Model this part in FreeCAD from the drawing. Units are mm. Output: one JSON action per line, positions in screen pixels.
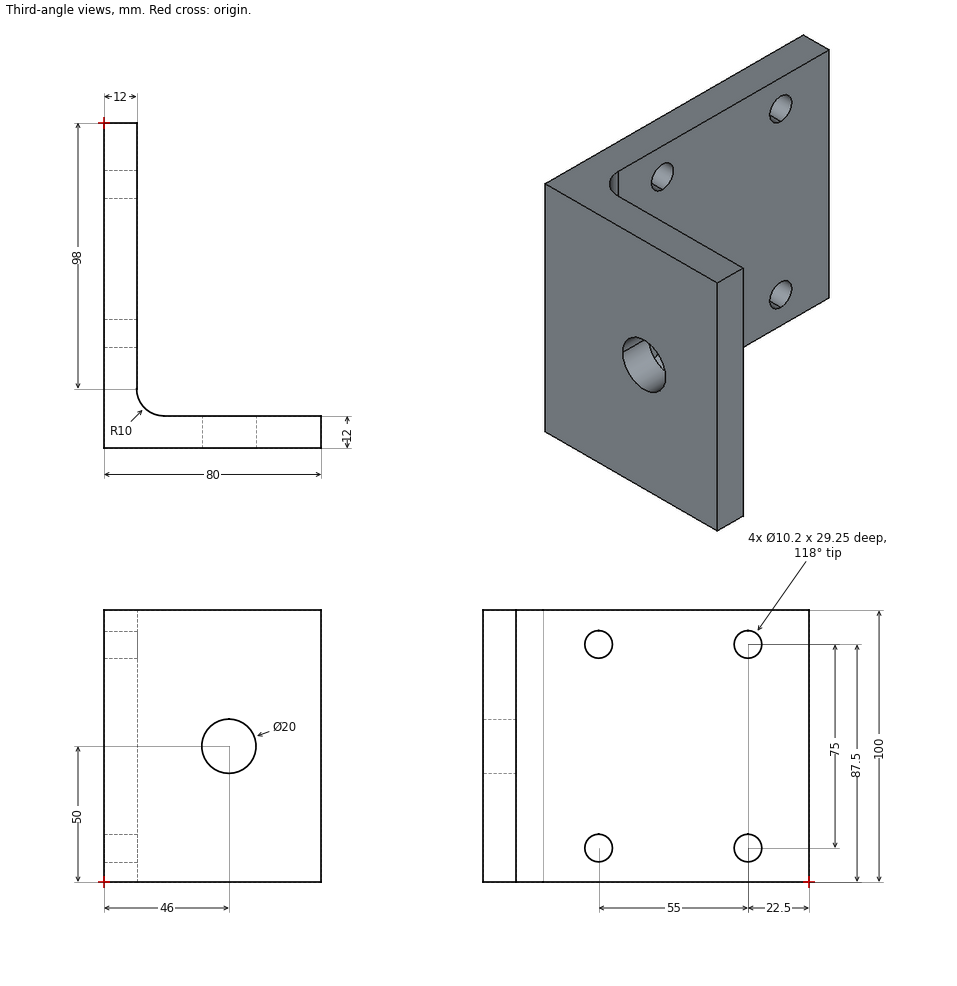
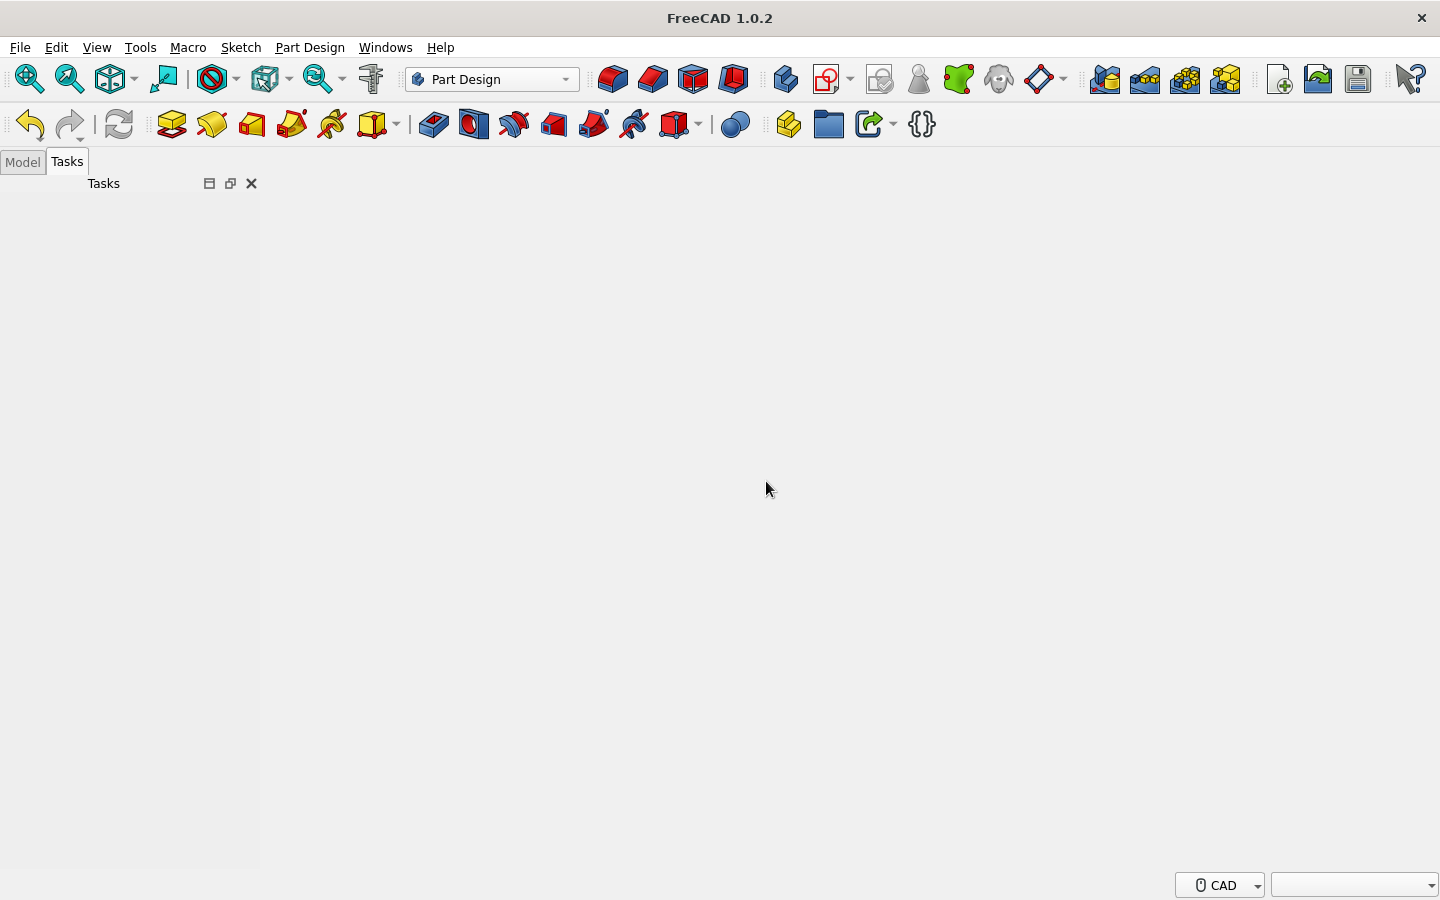
{"action": "left_click", "coordinate": [1278, 80]}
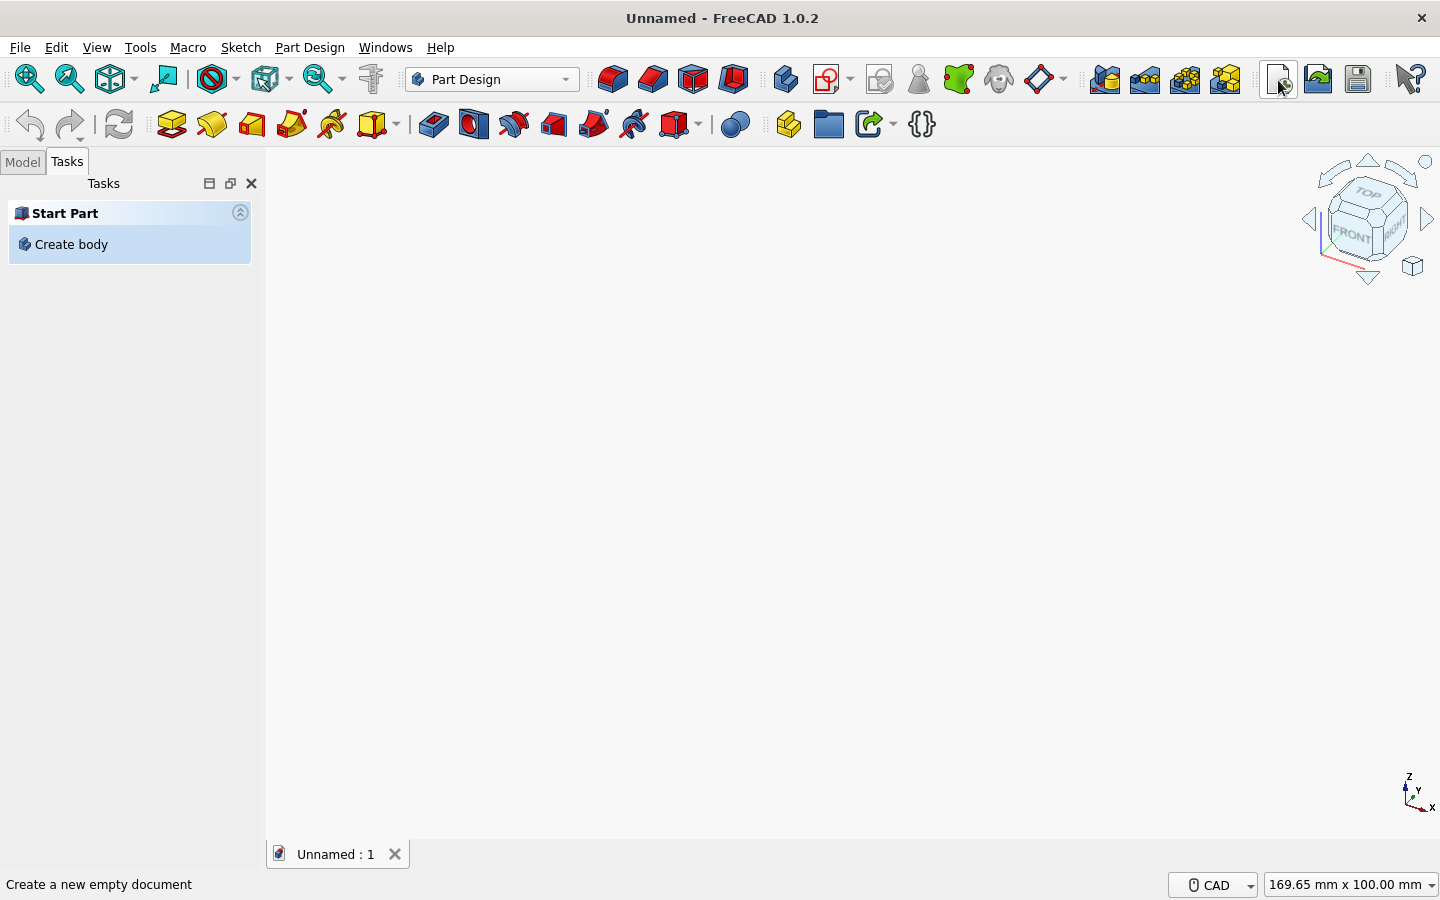
{"action": "left_click", "coordinate": [826, 80]}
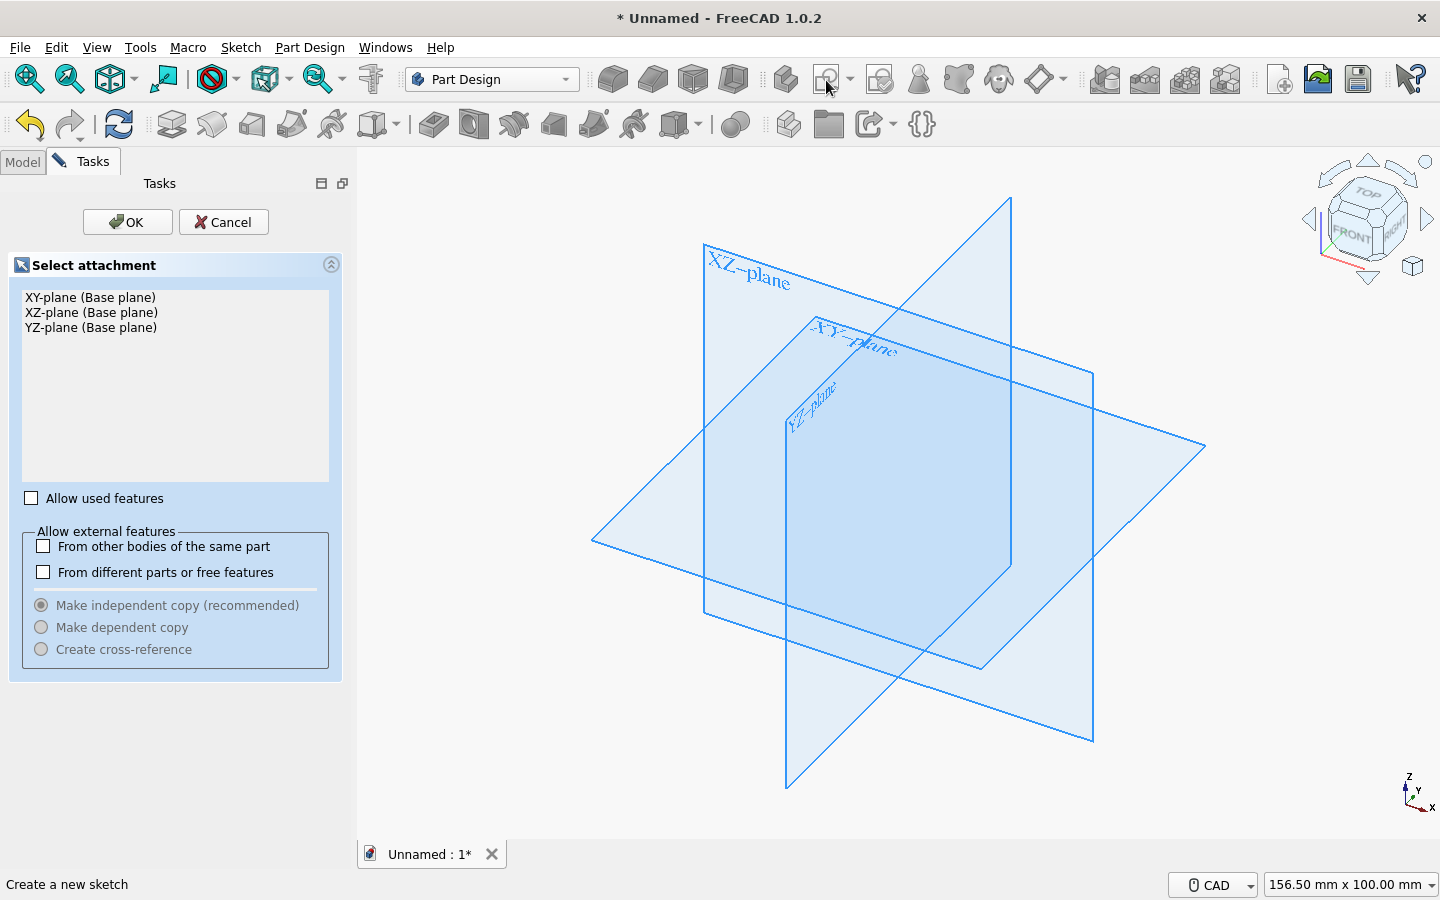
{"action": "left_click", "coordinate": [82, 298]}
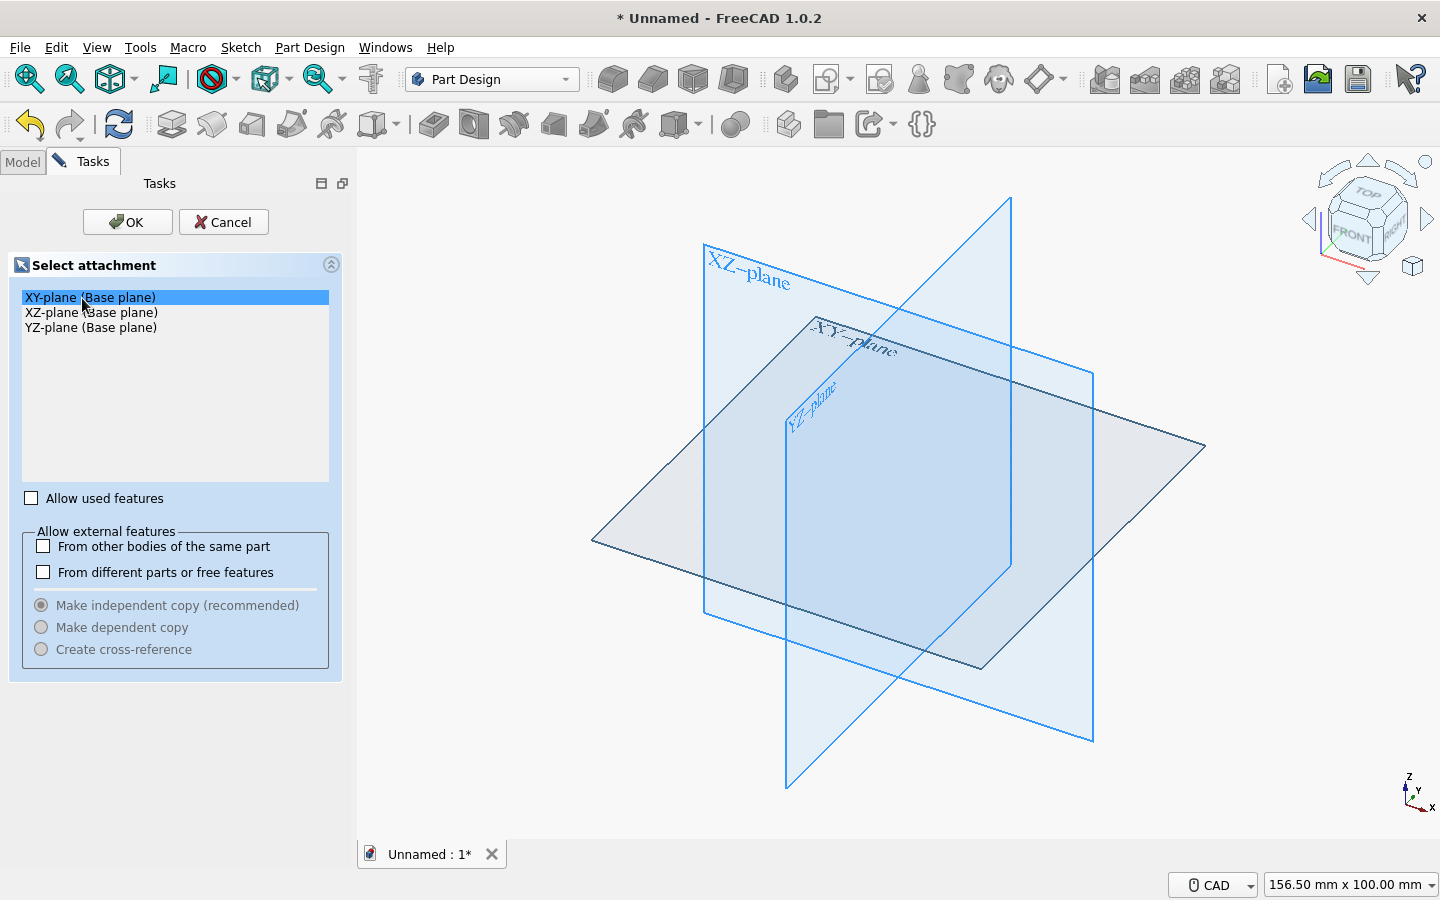
{"action": "left_click", "coordinate": [128, 222]}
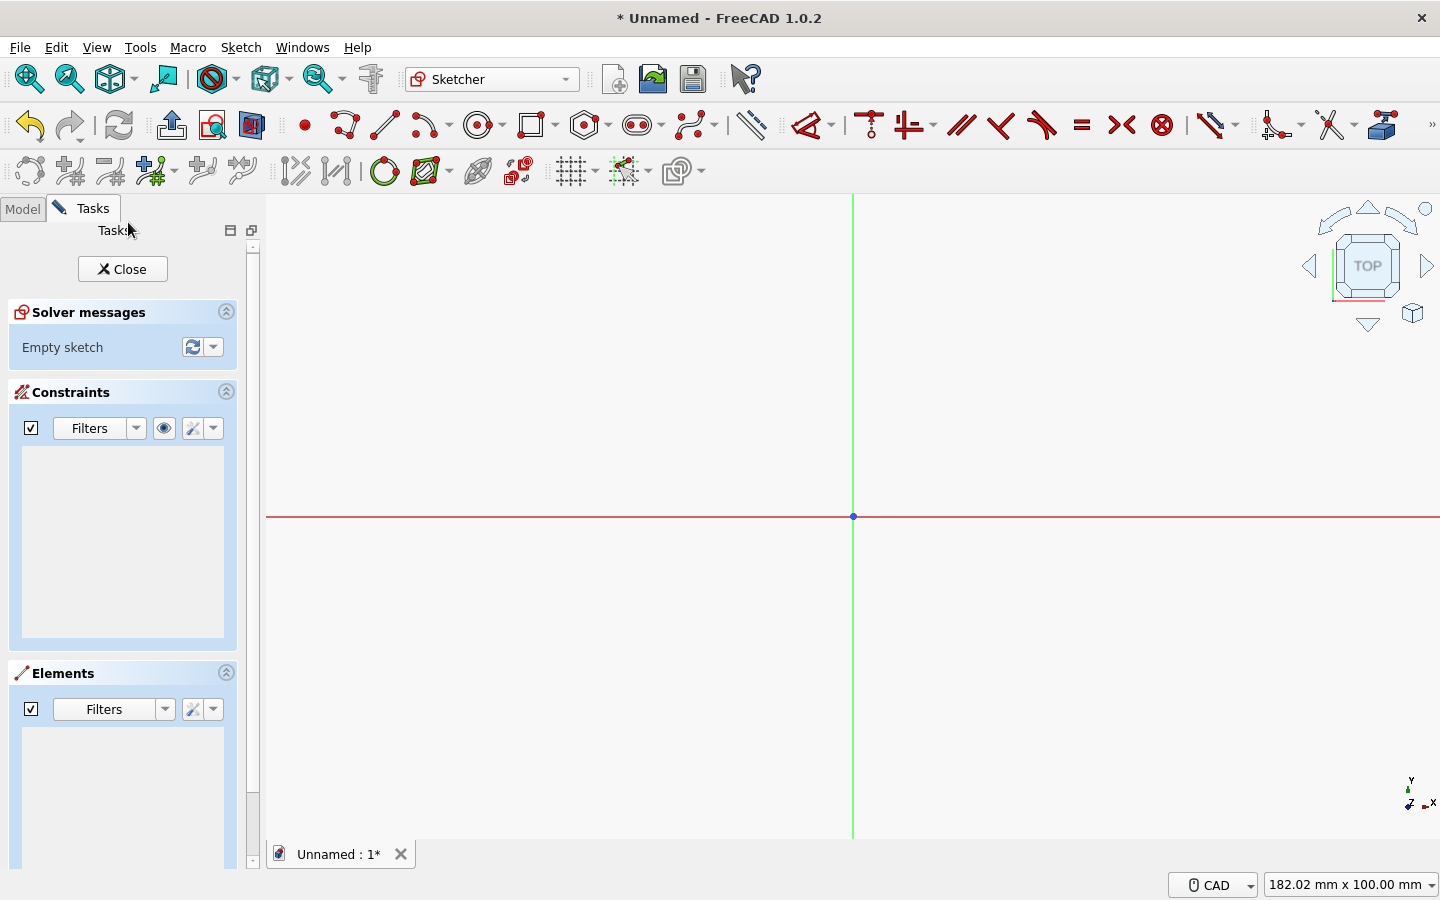
{"action": "scroll", "coordinate": [518, 222], "scroll_direction": "down", "scroll_amount": 4}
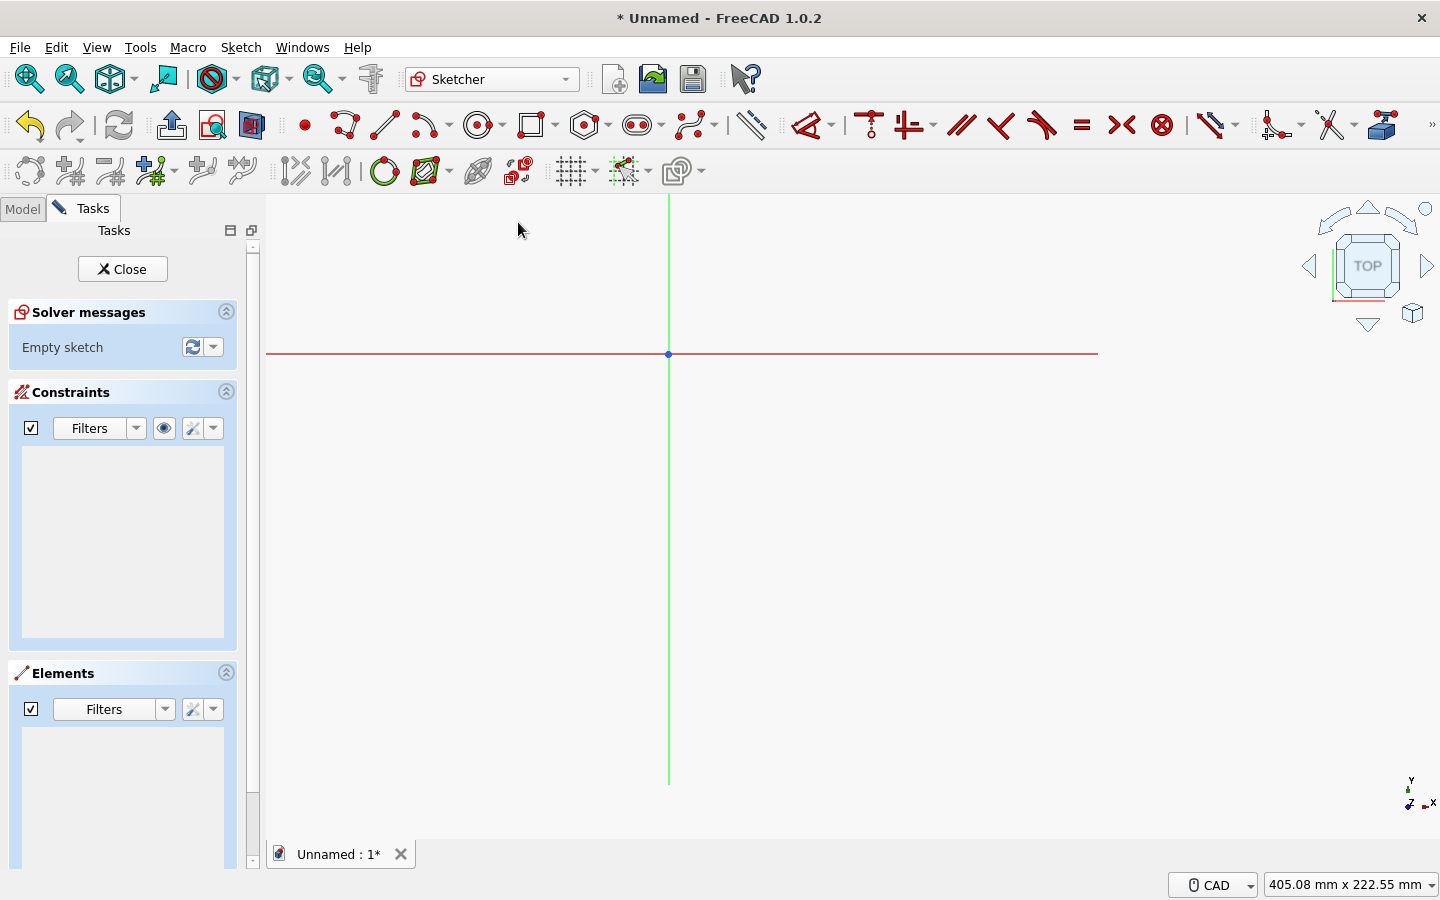
{"action": "key", "text": "g m"}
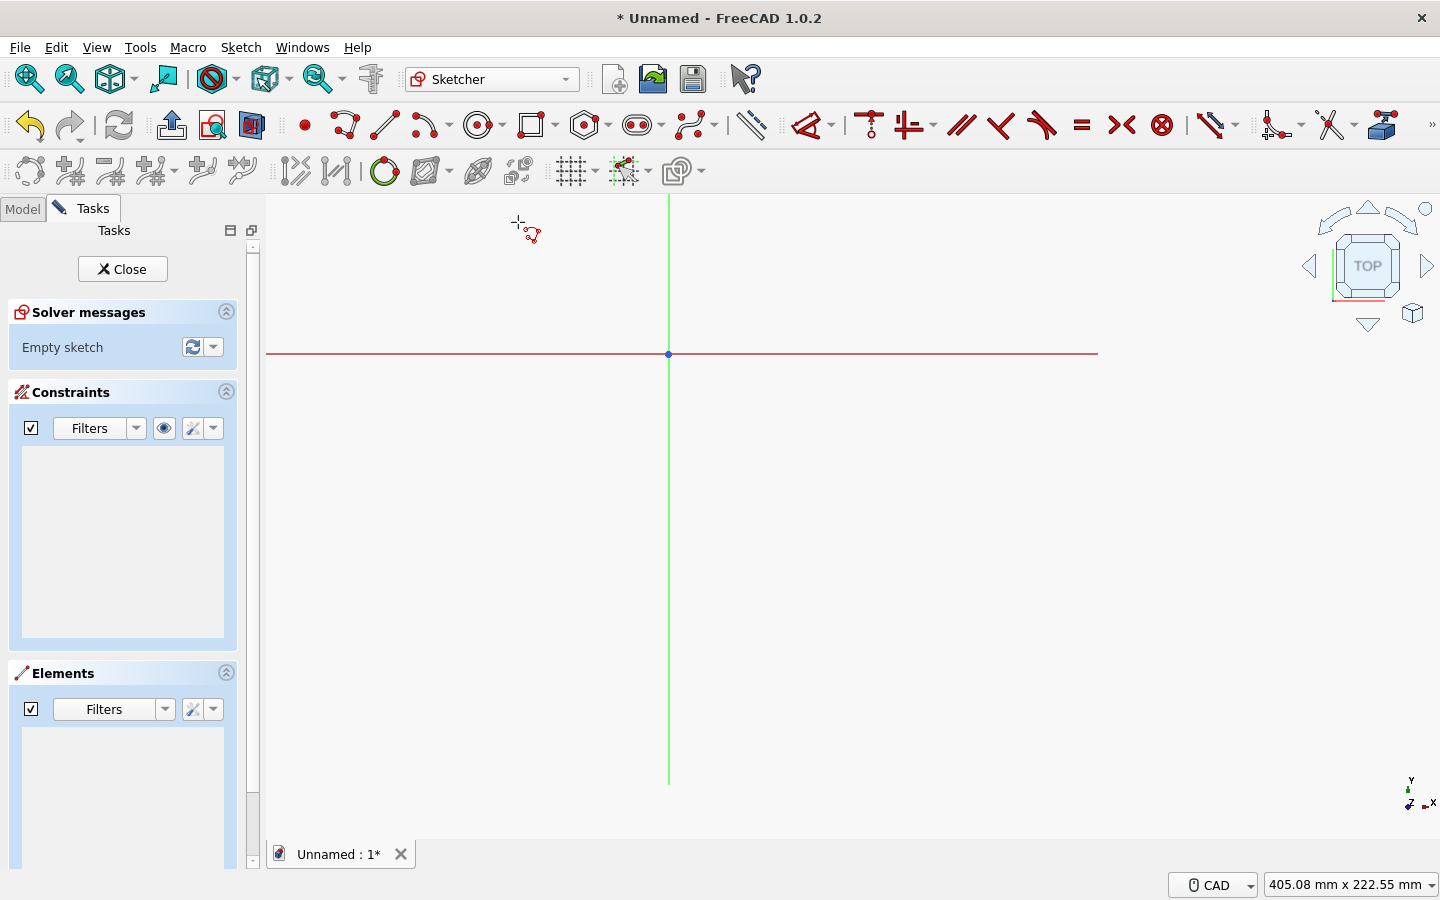
{"action": "left_click", "coordinate": [703, 638]}
{"action": "left_click", "coordinate": [703, 354]}
{"action": "left_click", "coordinate": [669, 354]}
{"action": "left_click", "coordinate": [678, 702]}
{"action": "left_click", "coordinate": [900, 702]}
{"action": "left_click", "coordinate": [900, 667]}
{"action": "left_click", "coordinate": [732, 667]}
{"action": "right_click", "coordinate": [732, 667]}